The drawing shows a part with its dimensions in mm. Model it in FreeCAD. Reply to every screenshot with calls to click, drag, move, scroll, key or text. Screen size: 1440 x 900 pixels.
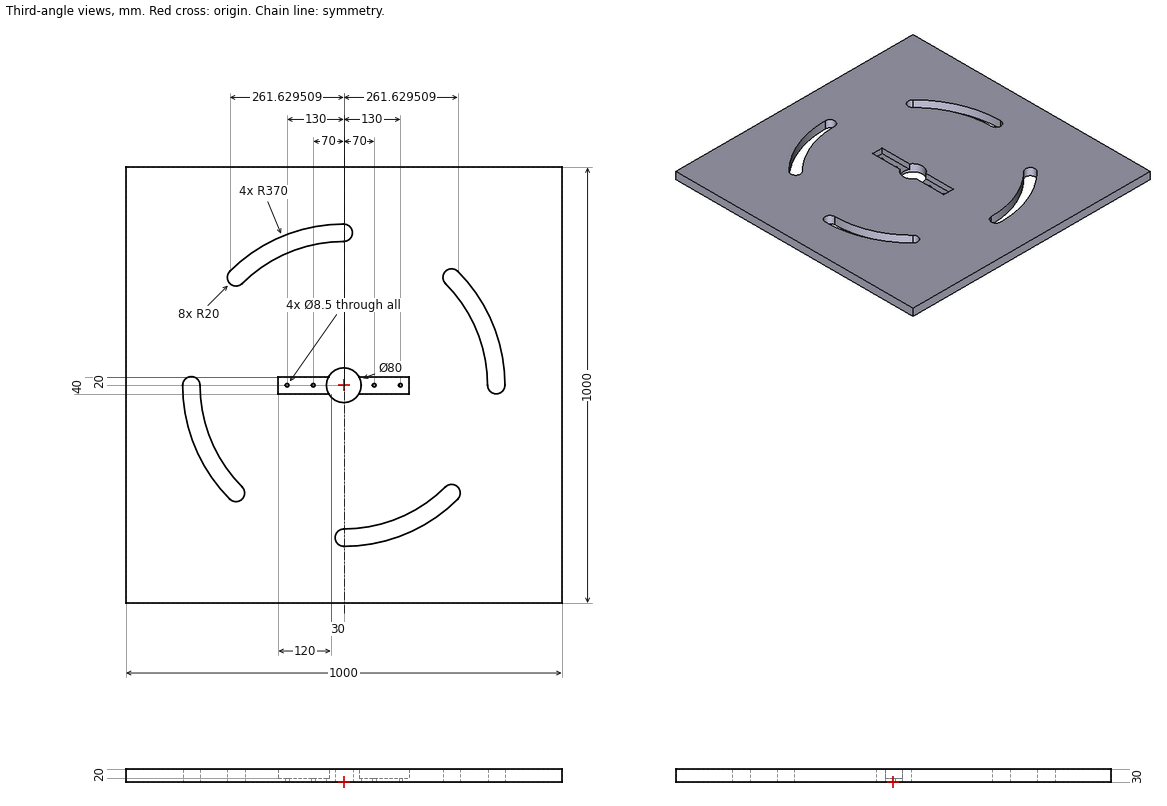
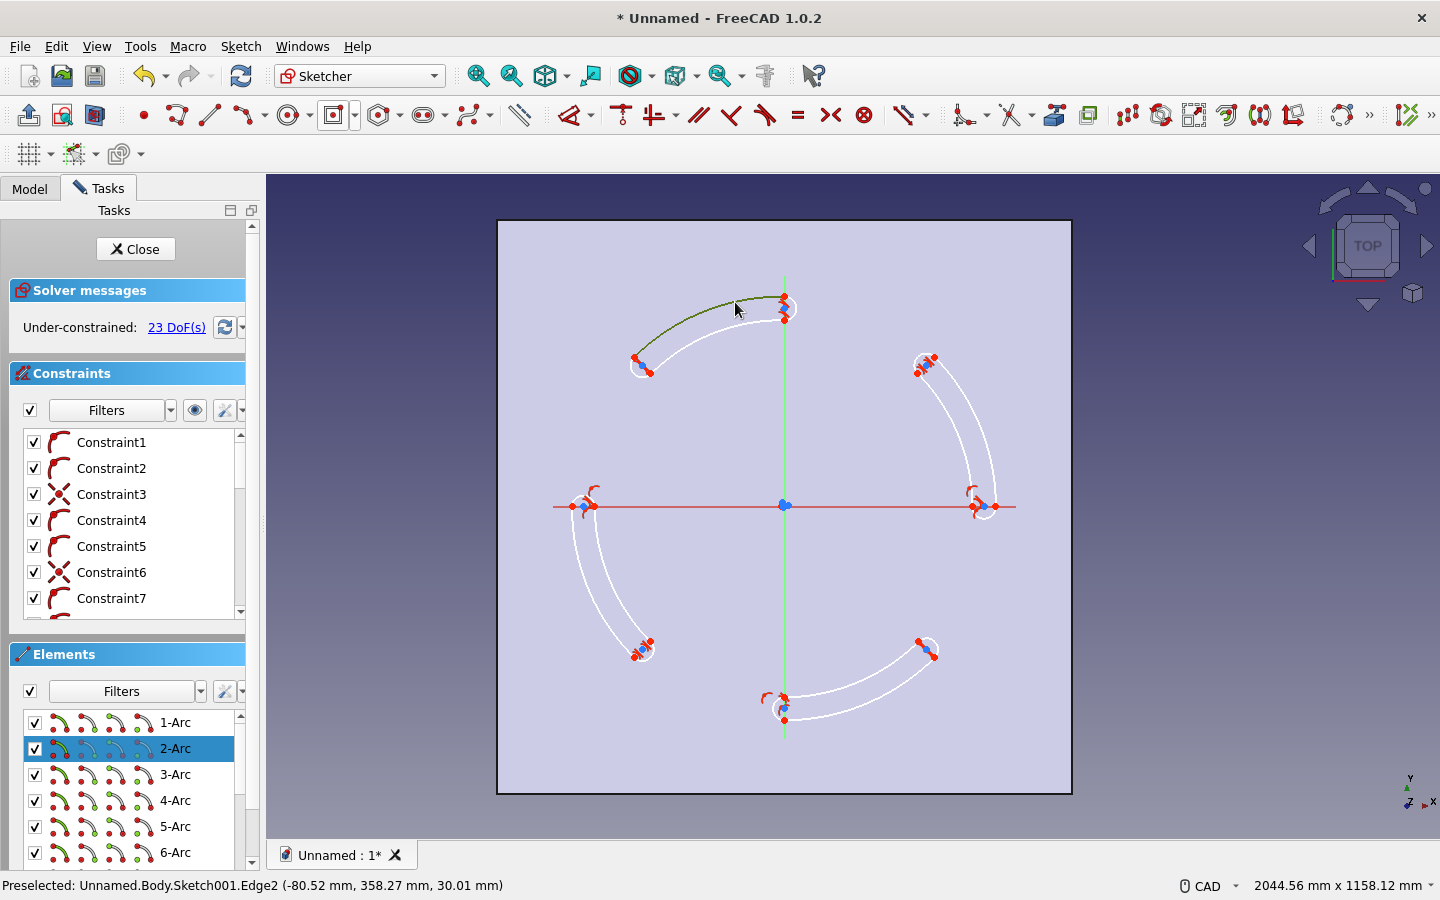
click(834, 714)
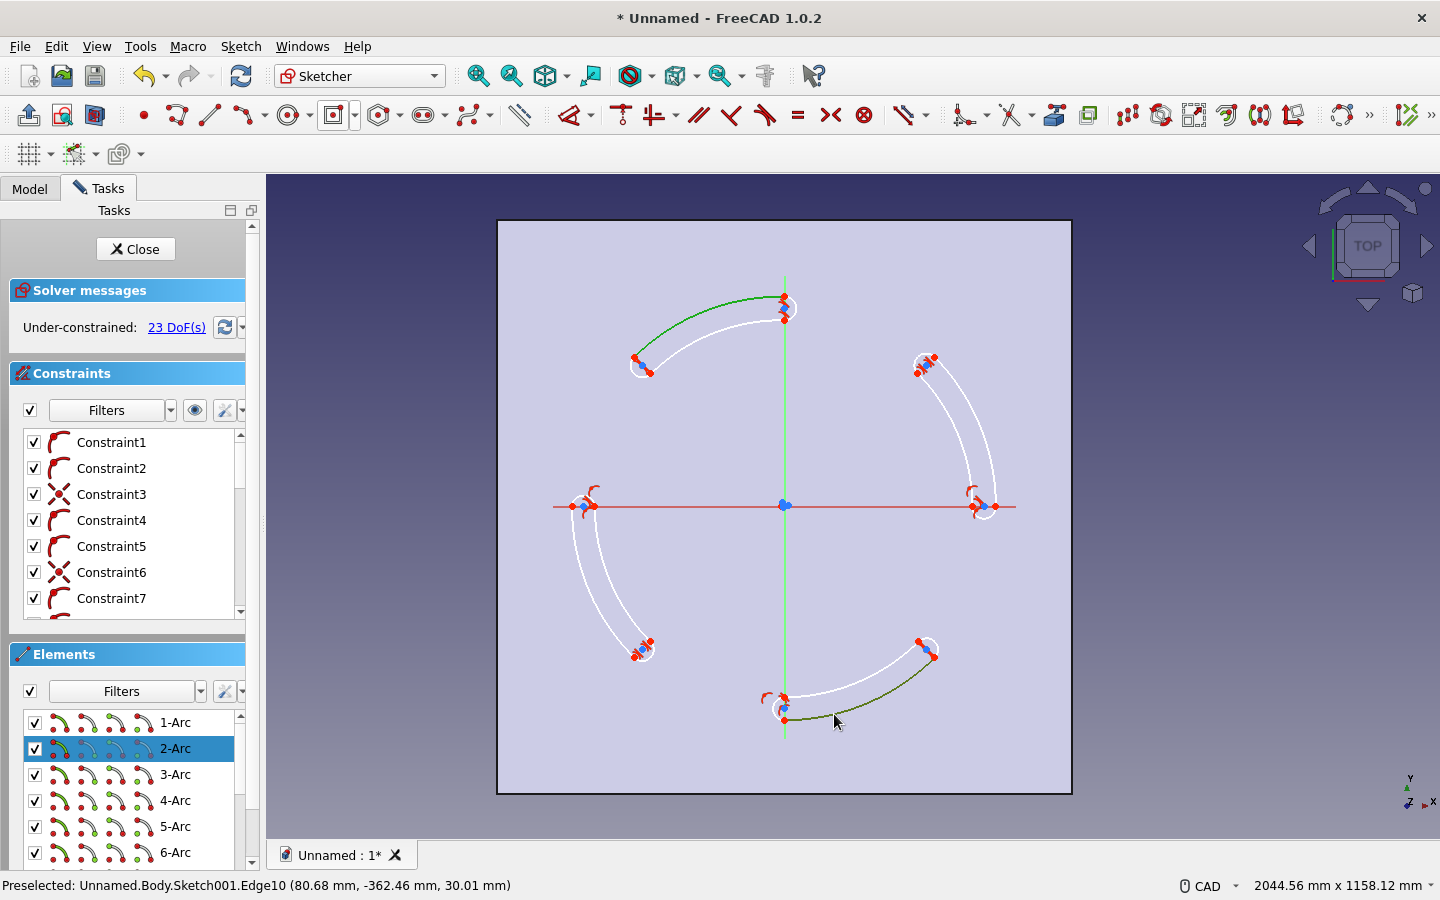
click(621, 116)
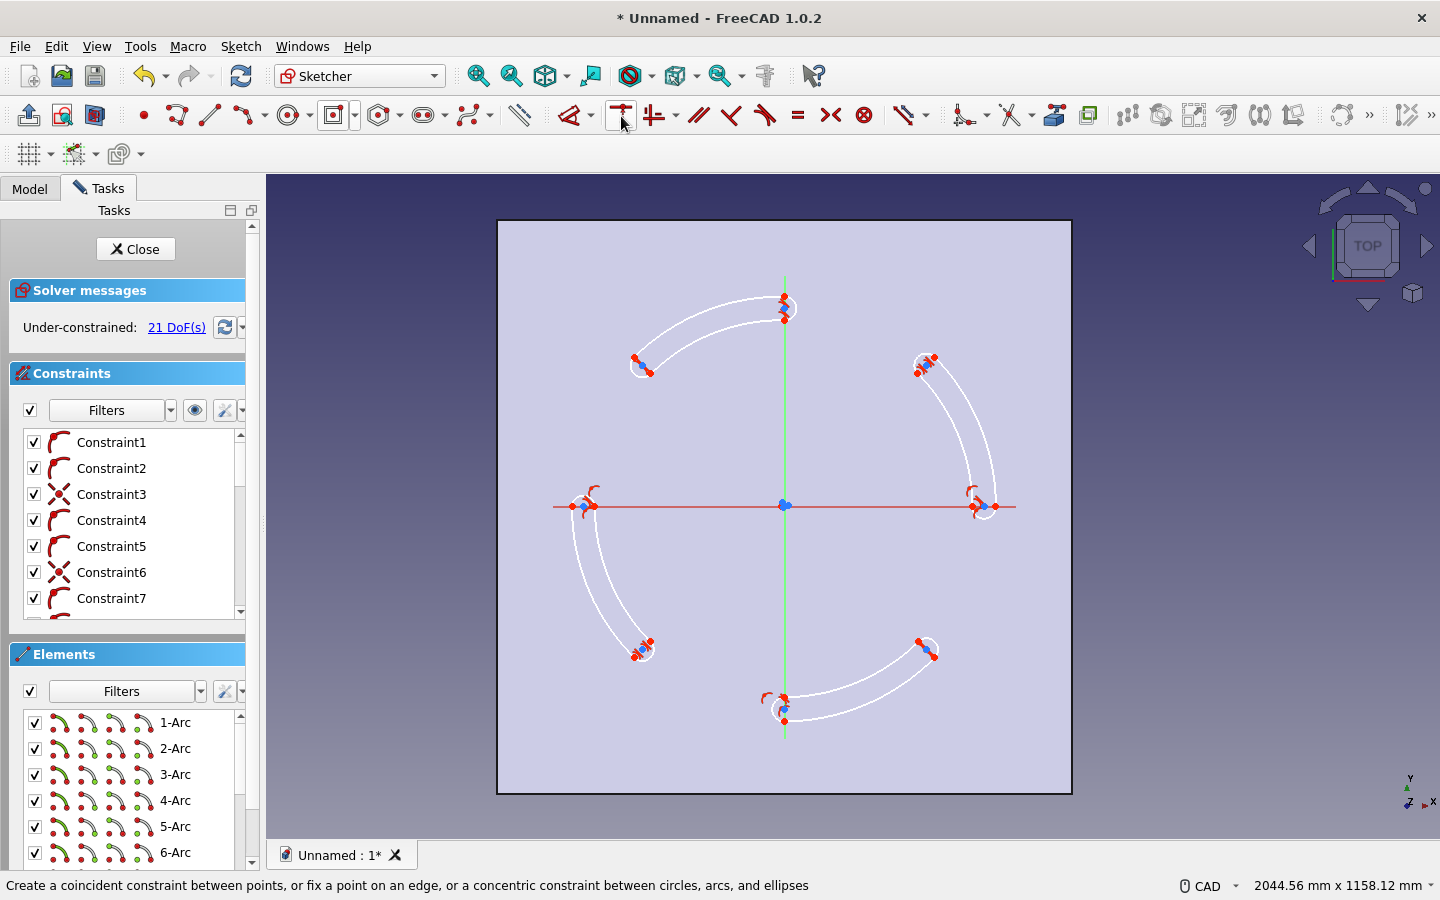
click(735, 302)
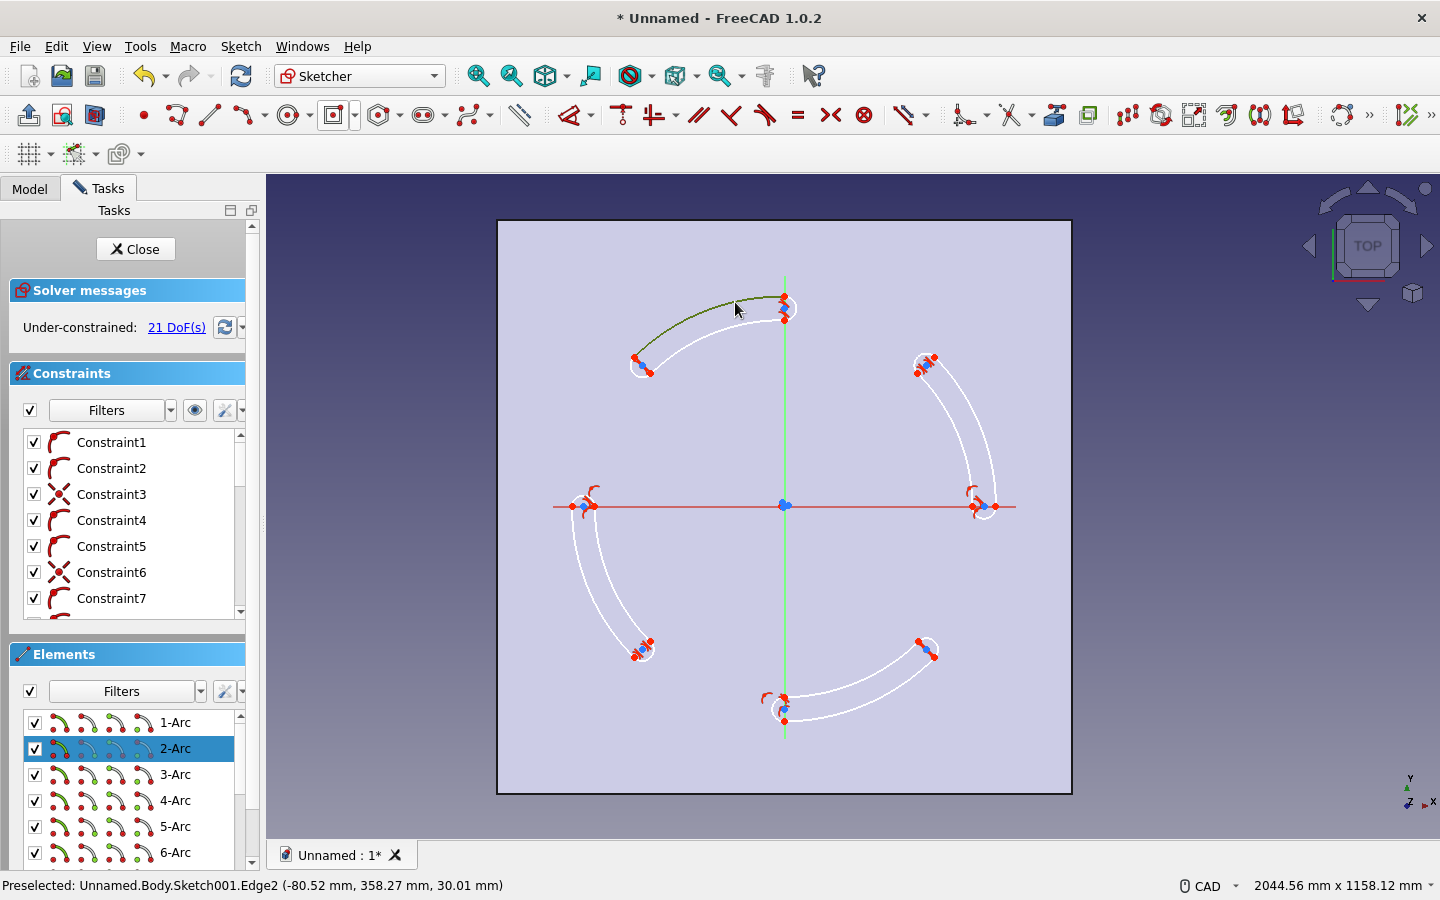
click(829, 692)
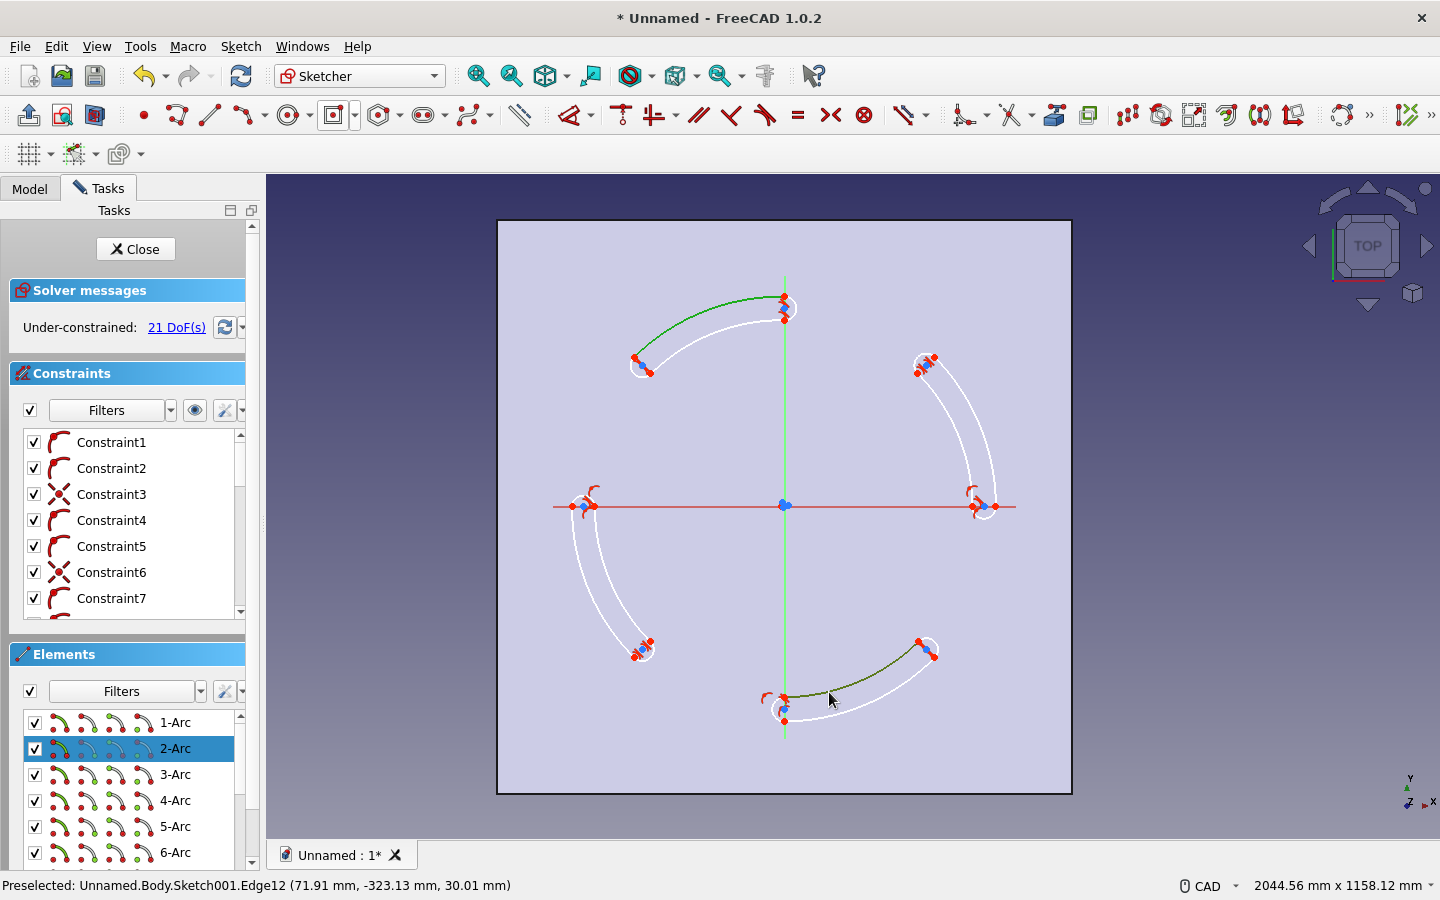
click(621, 116)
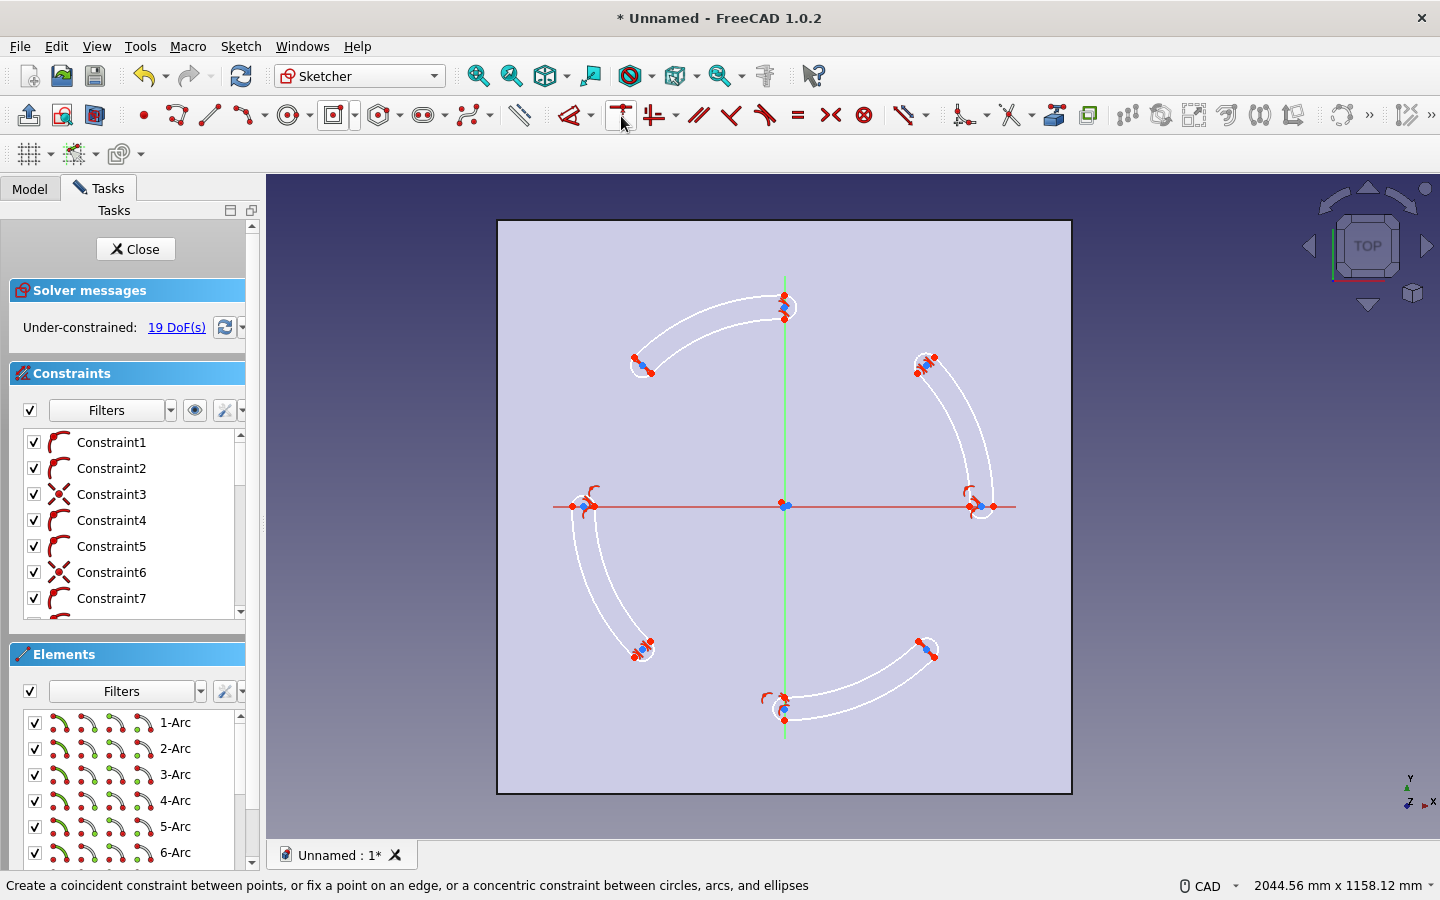
click(735, 301)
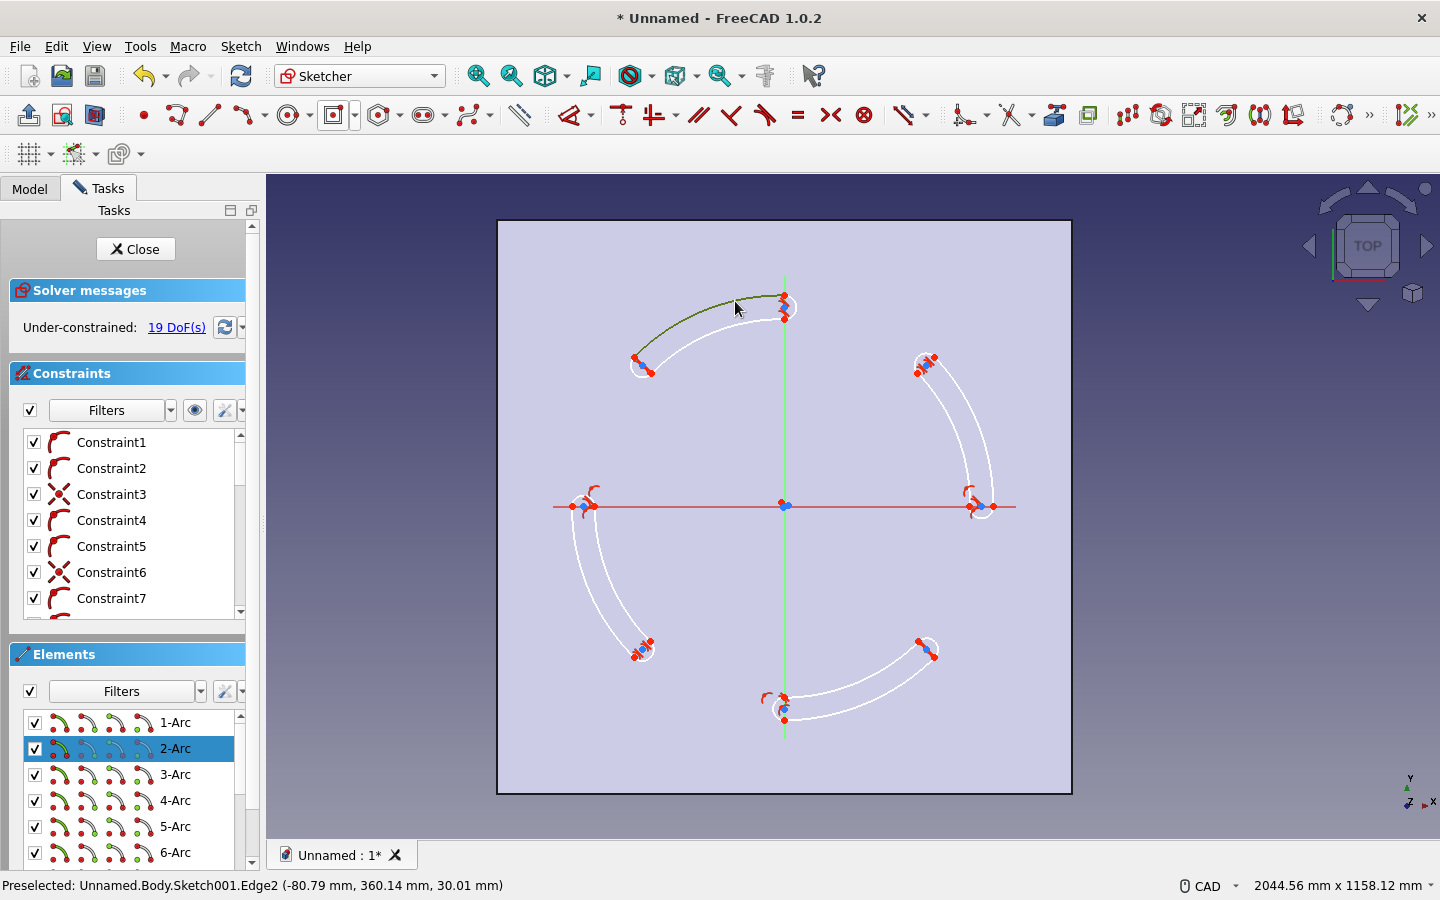
click(578, 557)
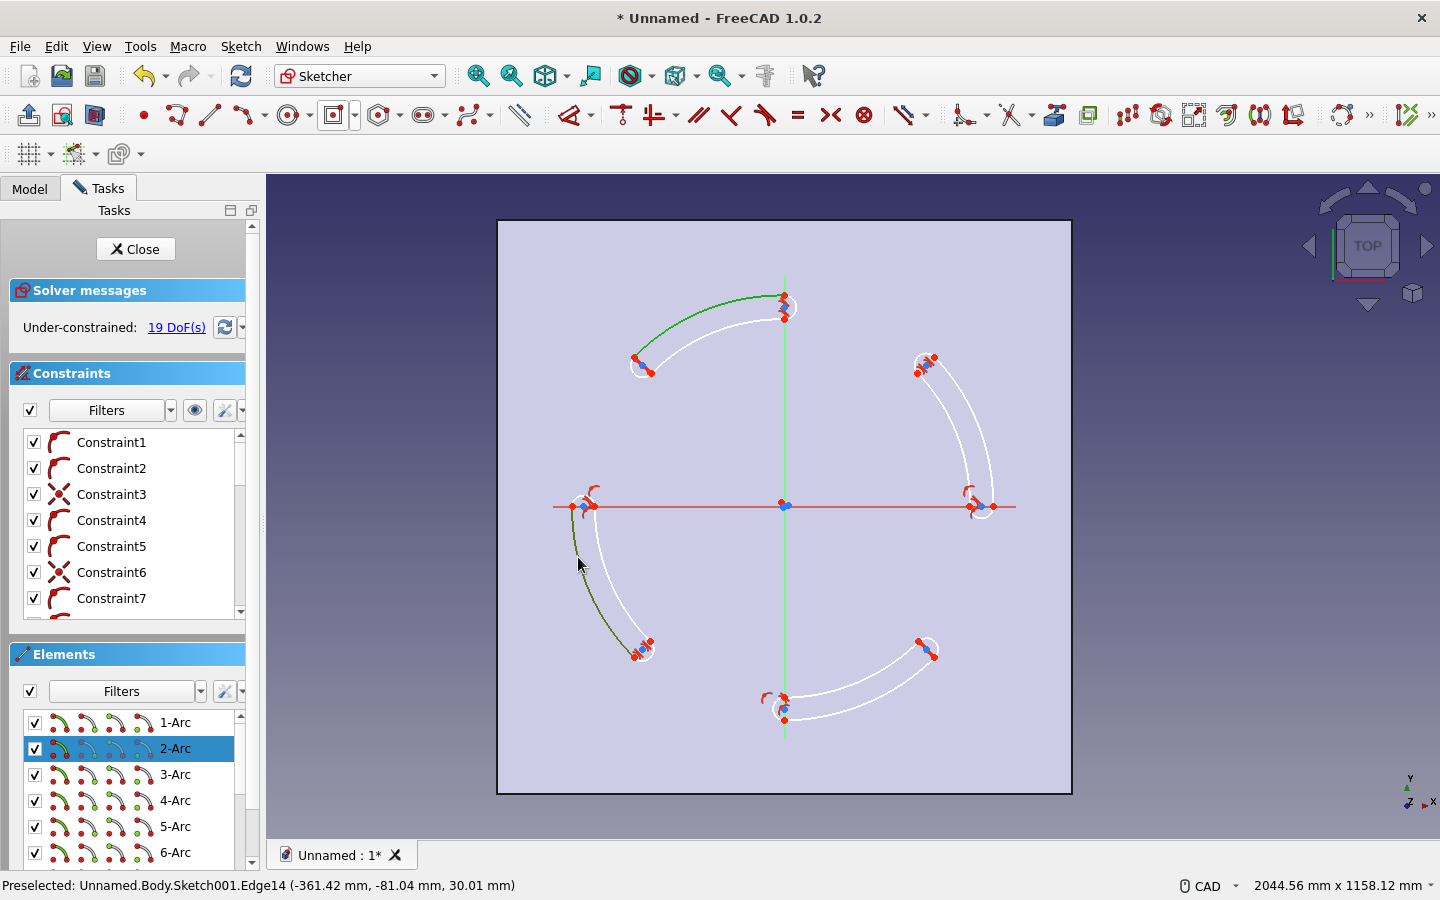
click(621, 116)